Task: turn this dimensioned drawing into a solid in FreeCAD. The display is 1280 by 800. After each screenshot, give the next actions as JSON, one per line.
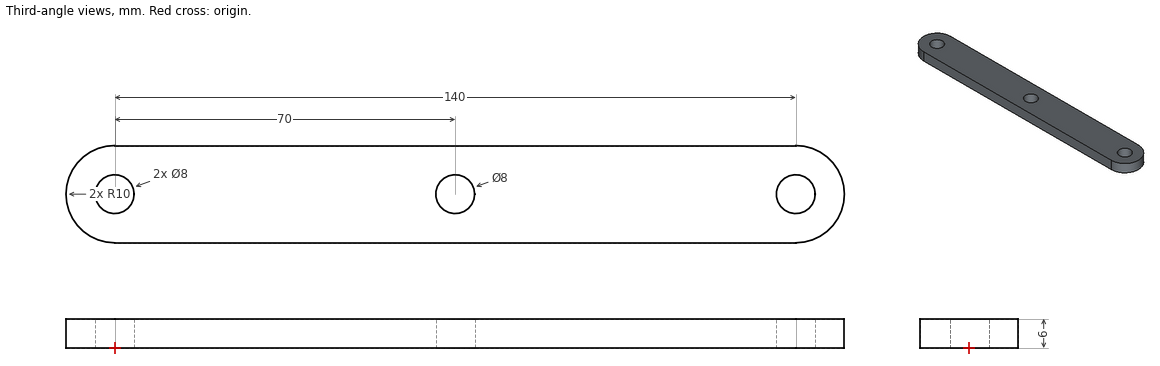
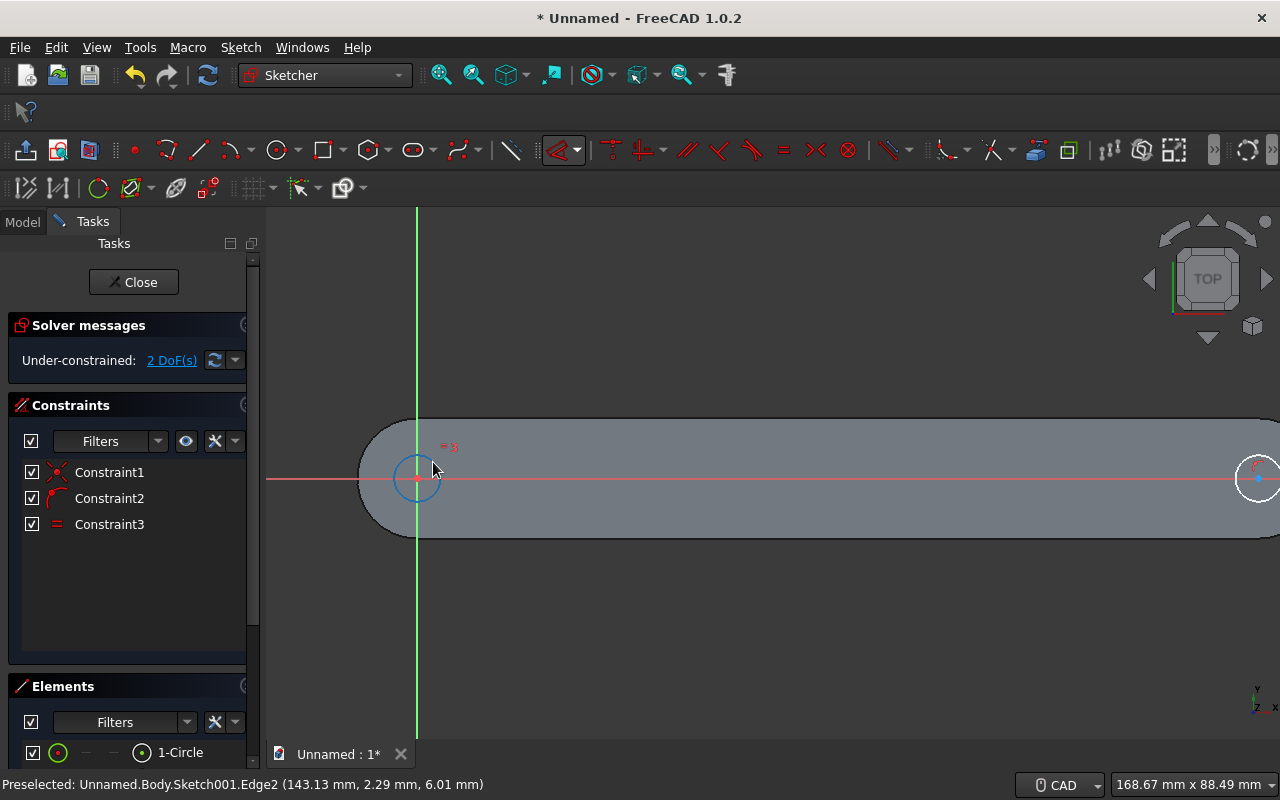
{"action": "left_click", "coordinate": [434, 462]}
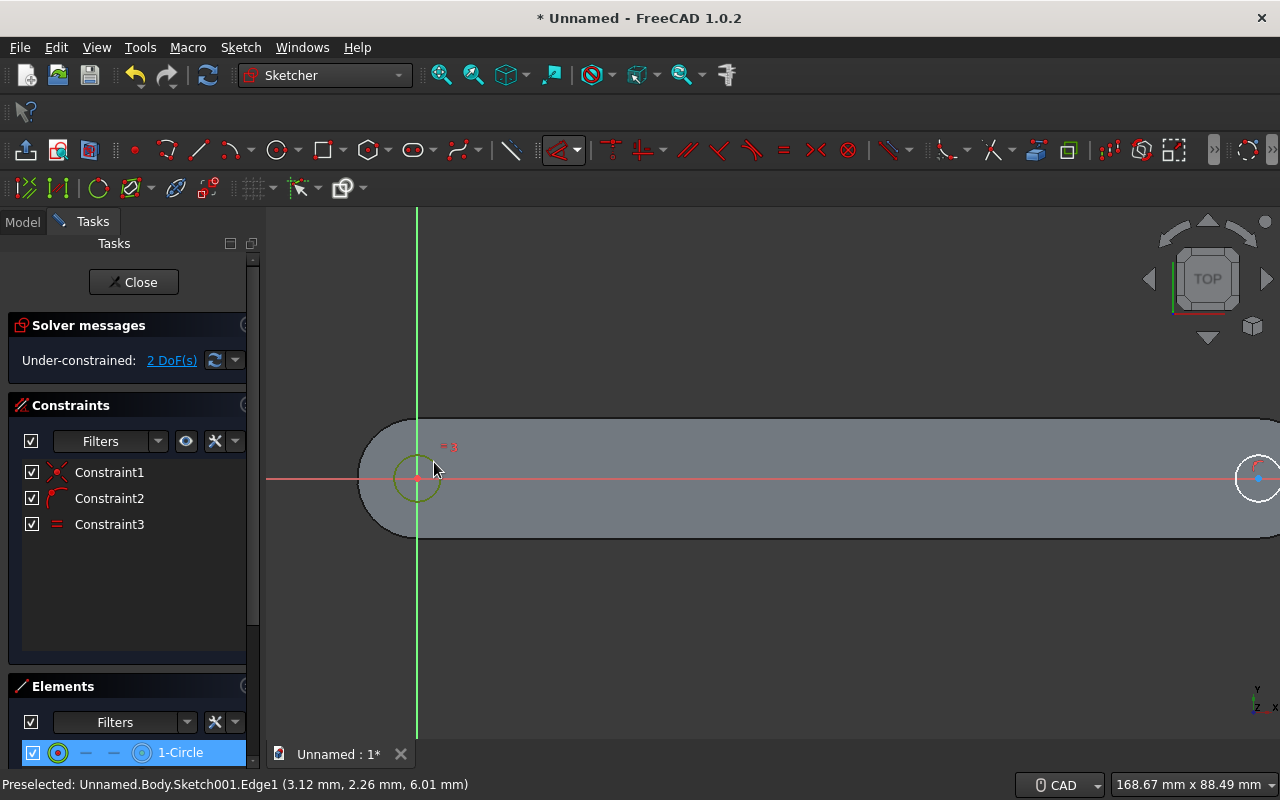
{"action": "key", "text": "k o"}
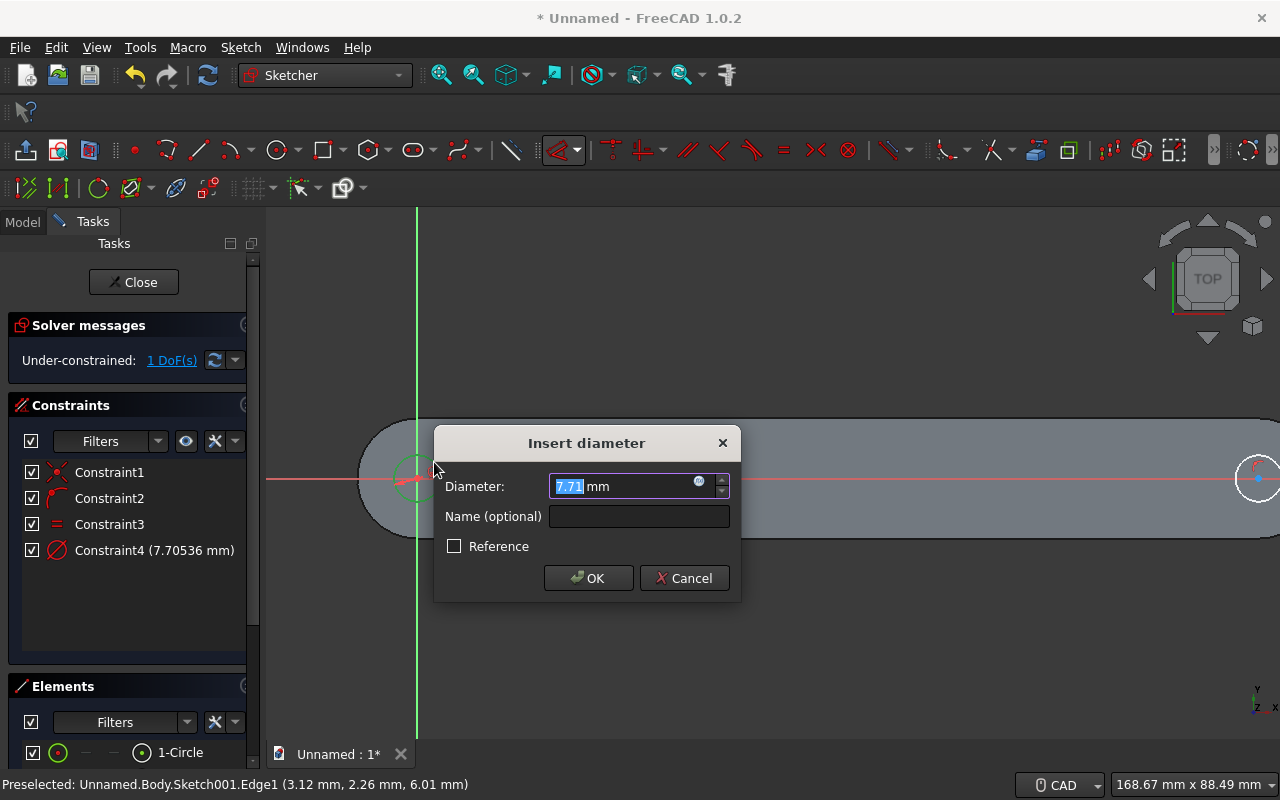
{"action": "type", "text": "8"}
{"action": "key", "text": "Return"}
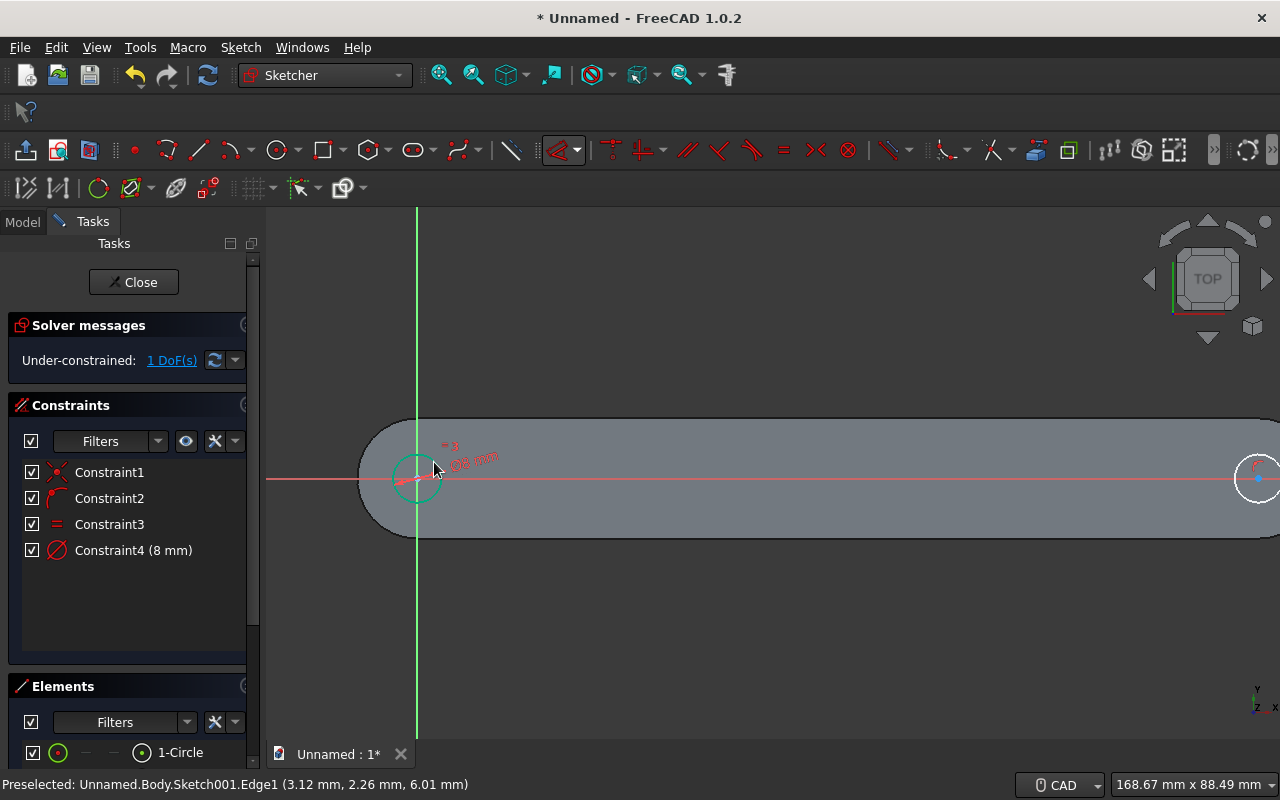
{"action": "scroll", "coordinate": [433, 462], "scroll_direction": "down", "scroll_amount": 2}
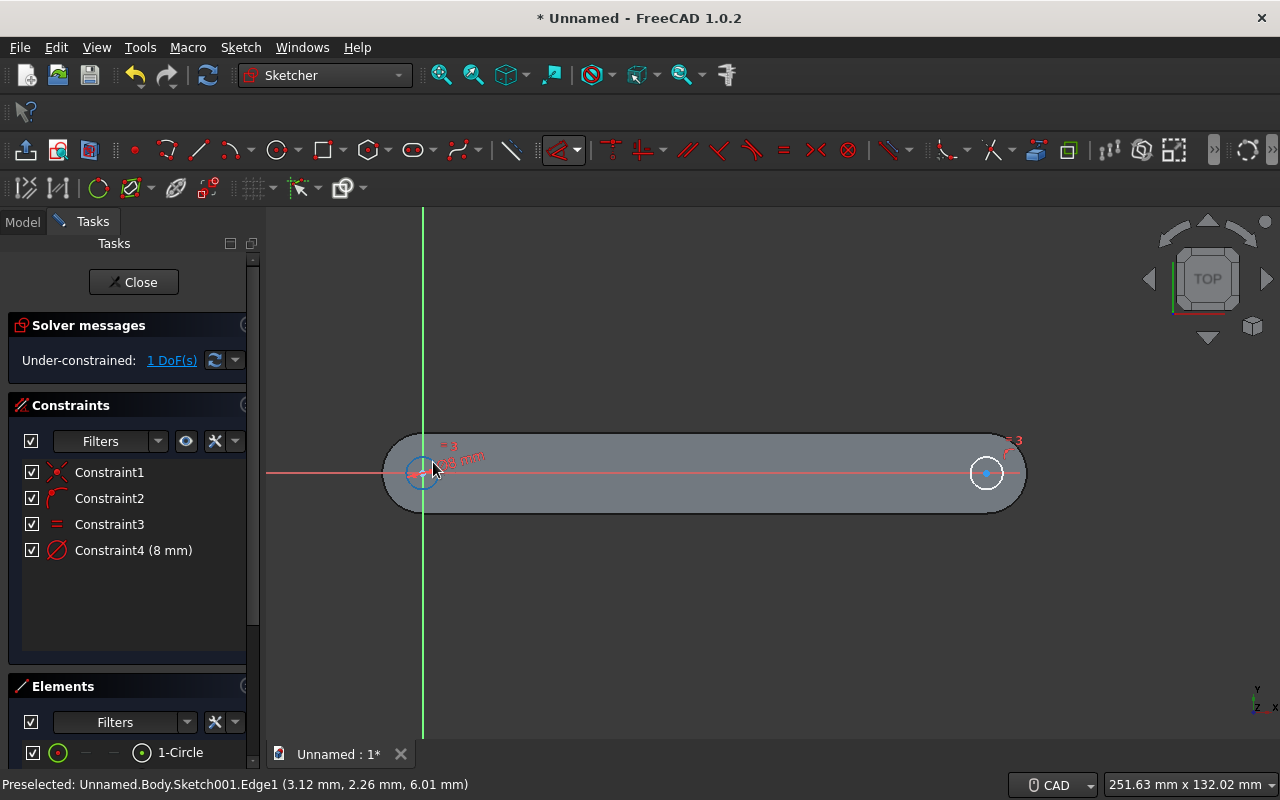
{"action": "left_click", "coordinate": [987, 473]}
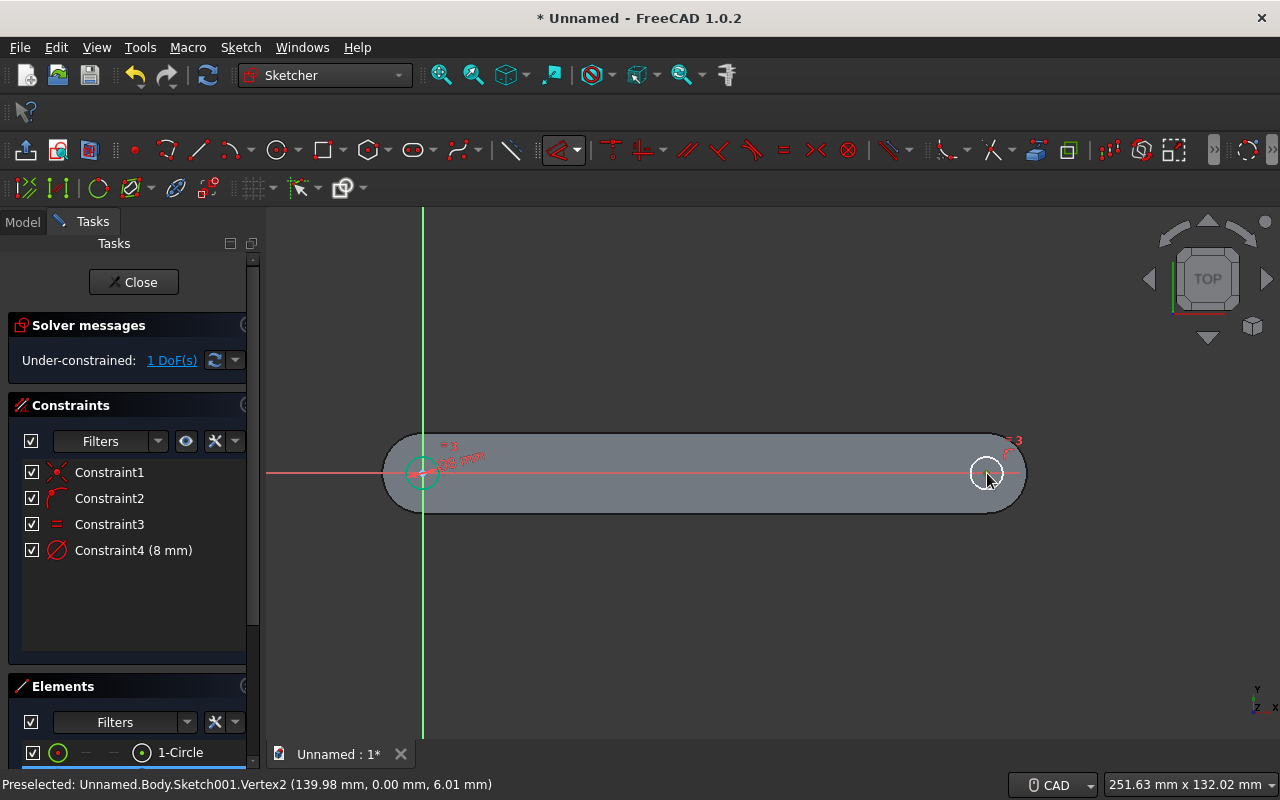
{"action": "key", "text": "l"}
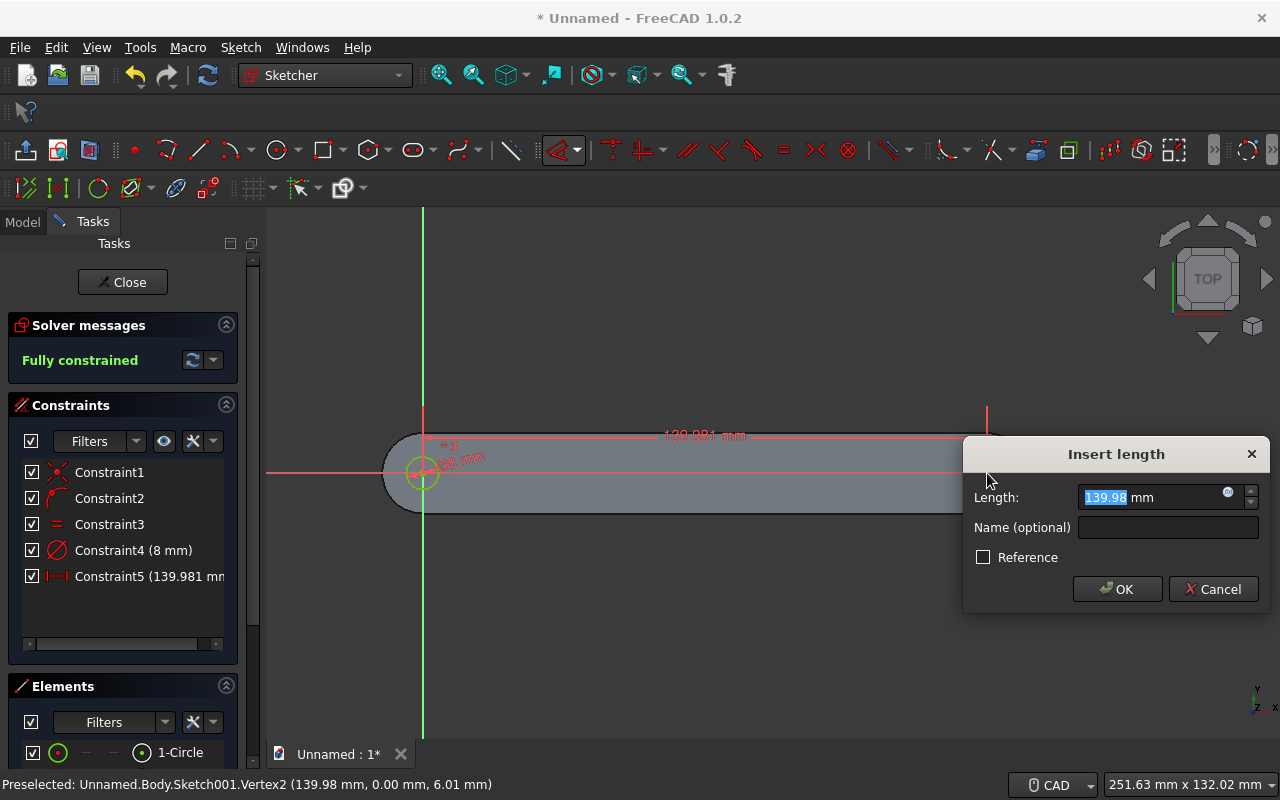
{"action": "type", "text": "140"}
{"action": "key", "text": "Return"}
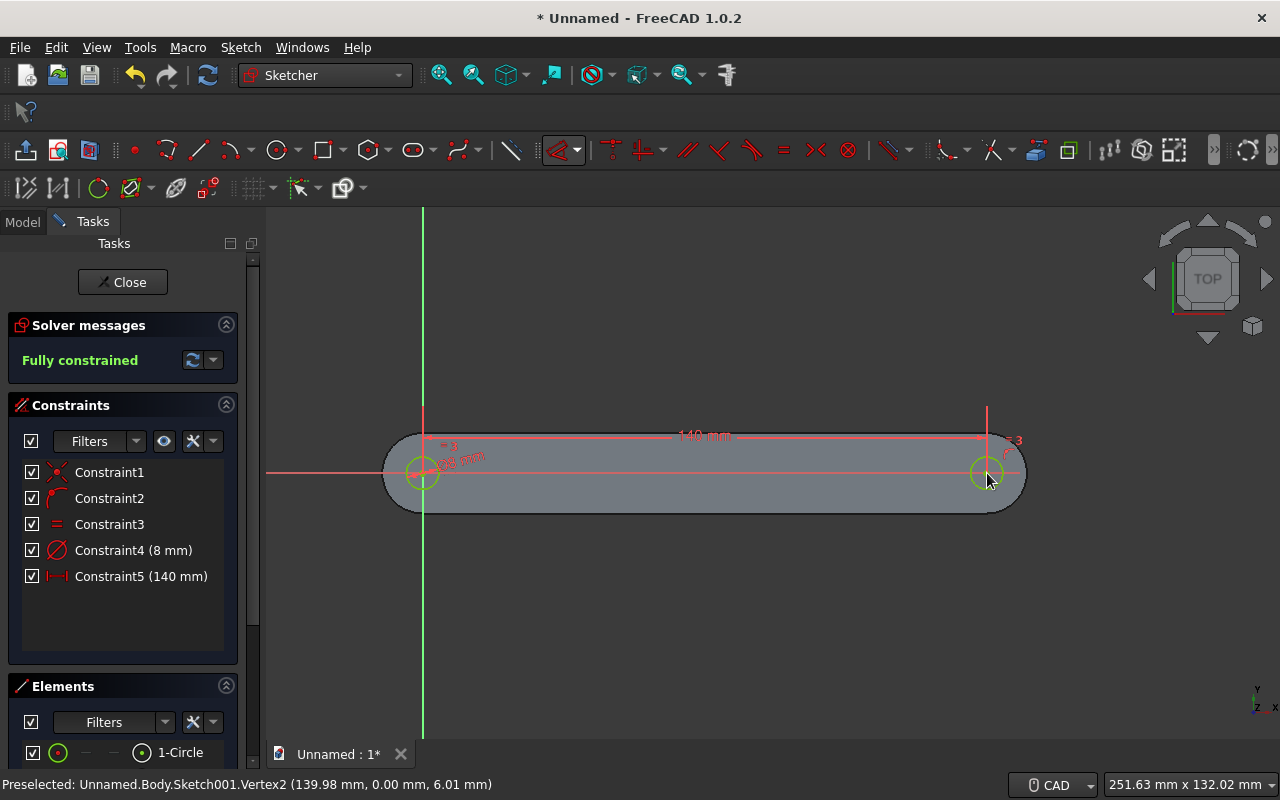
{"action": "left_click", "coordinate": [123, 282]}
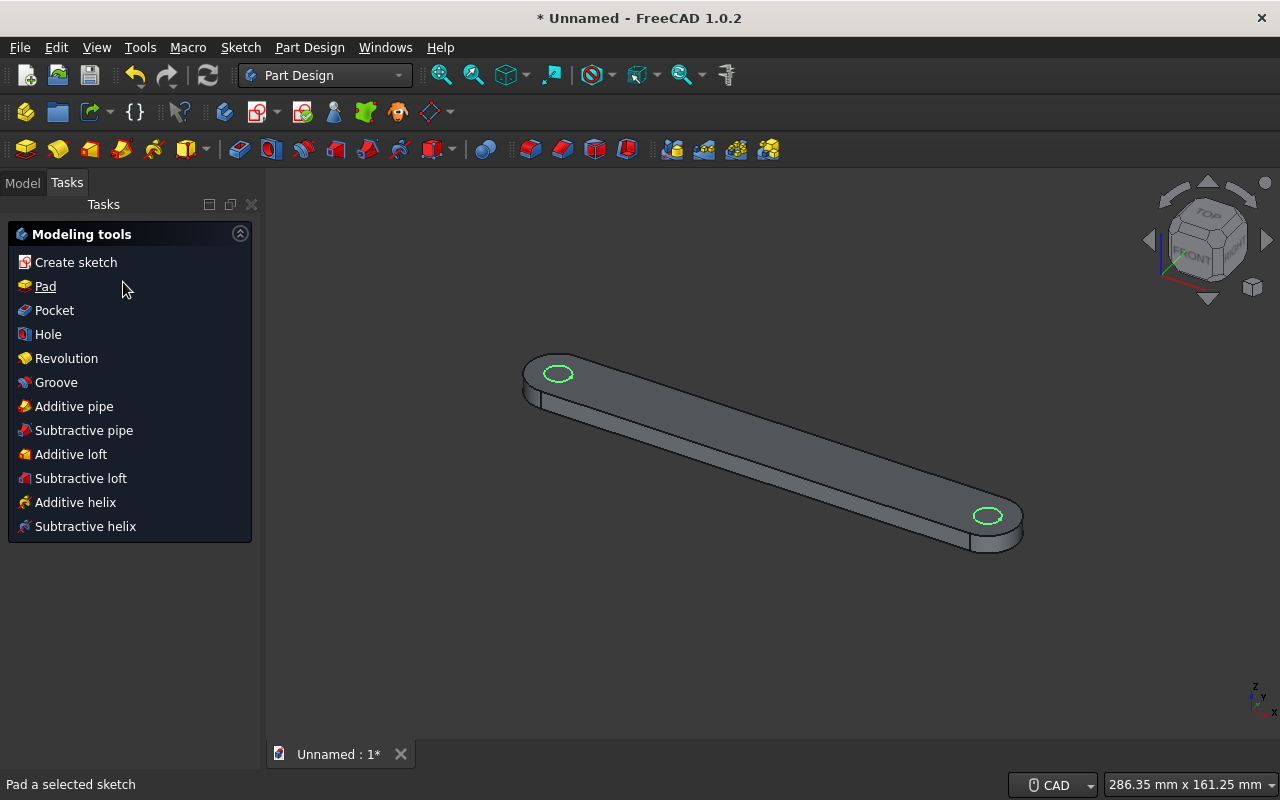
{"action": "left_click", "coordinate": [240, 150]}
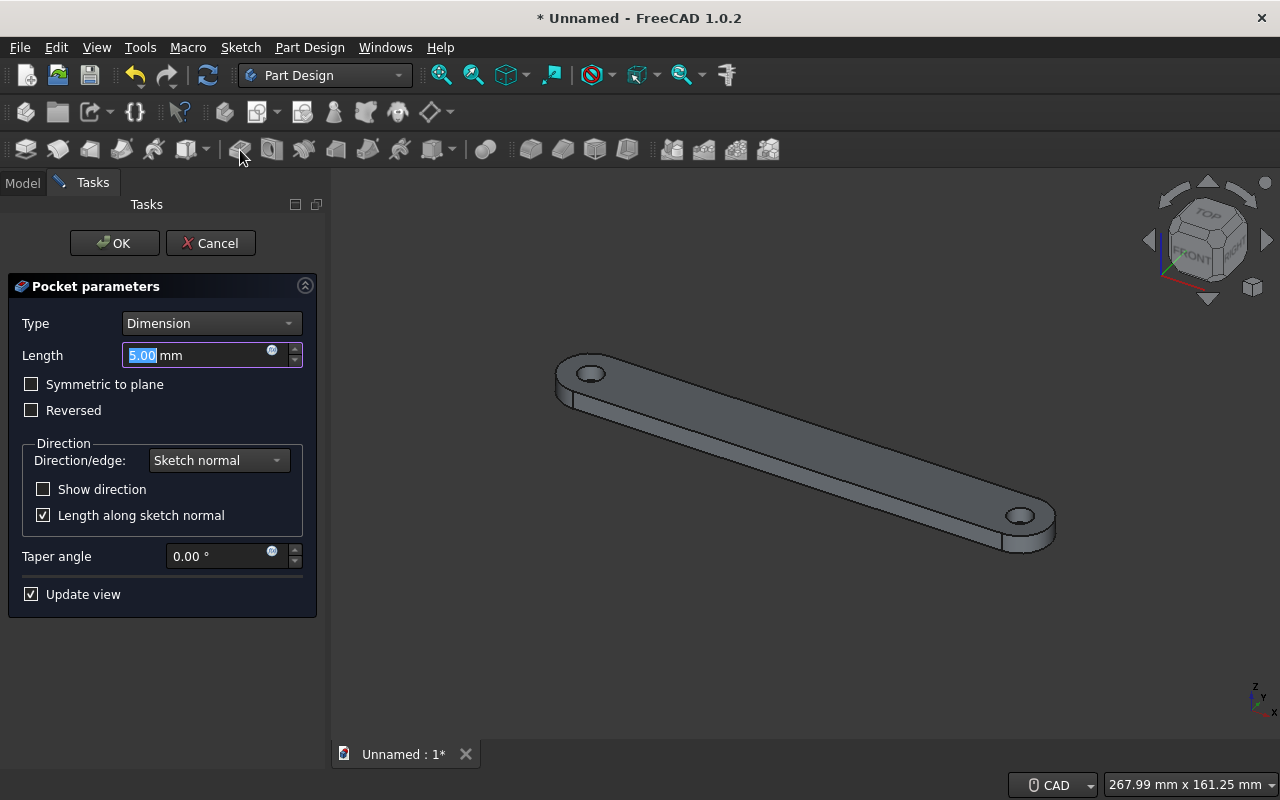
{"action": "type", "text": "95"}
{"action": "key", "text": "Tab"}